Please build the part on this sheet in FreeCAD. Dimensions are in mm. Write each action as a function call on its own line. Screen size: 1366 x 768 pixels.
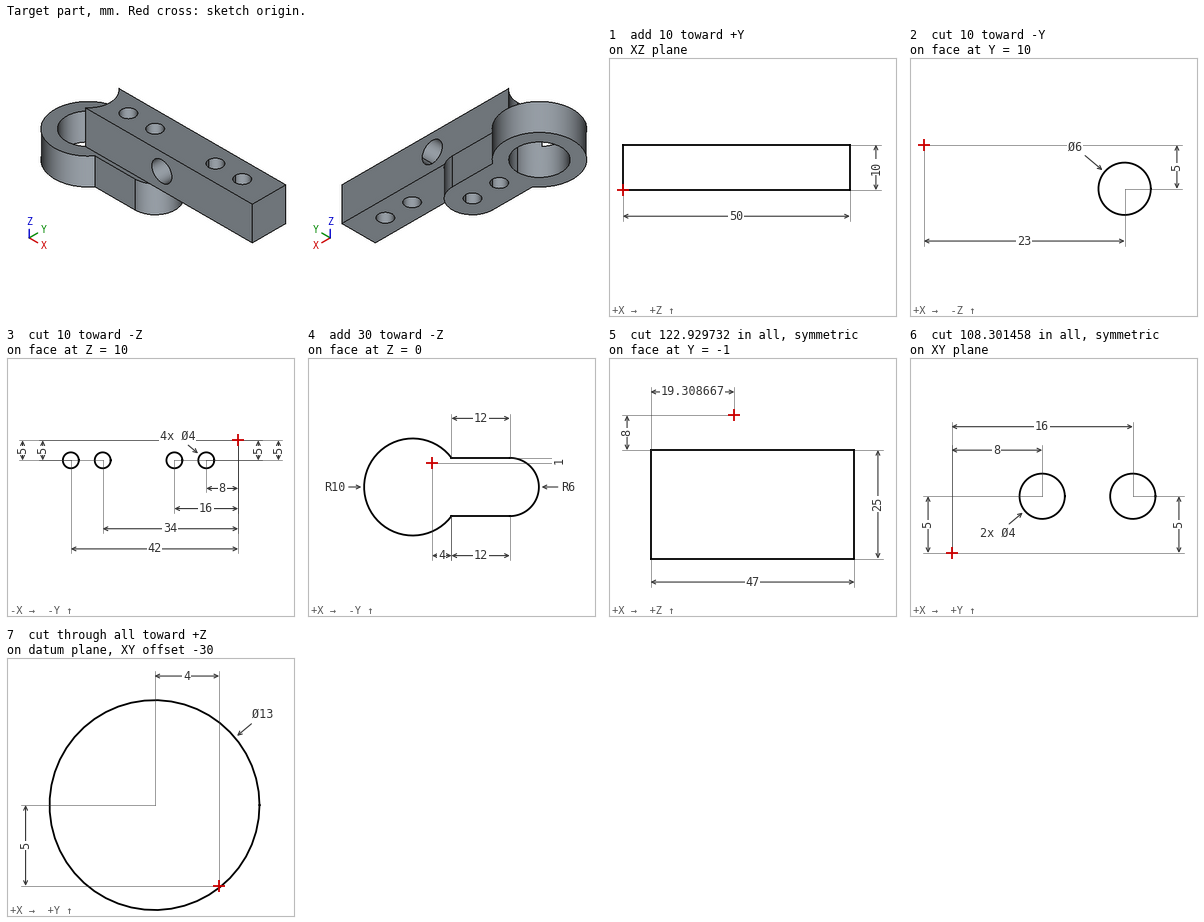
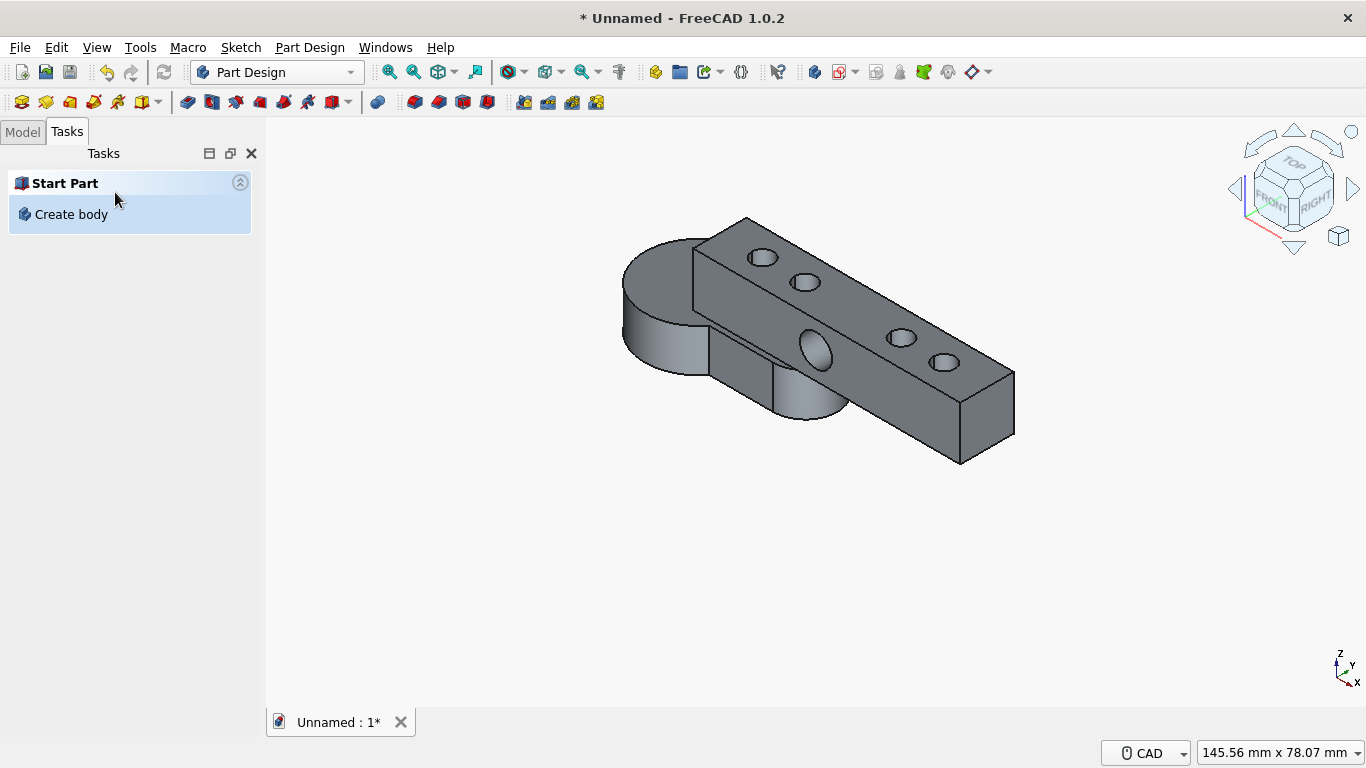
click(840, 72)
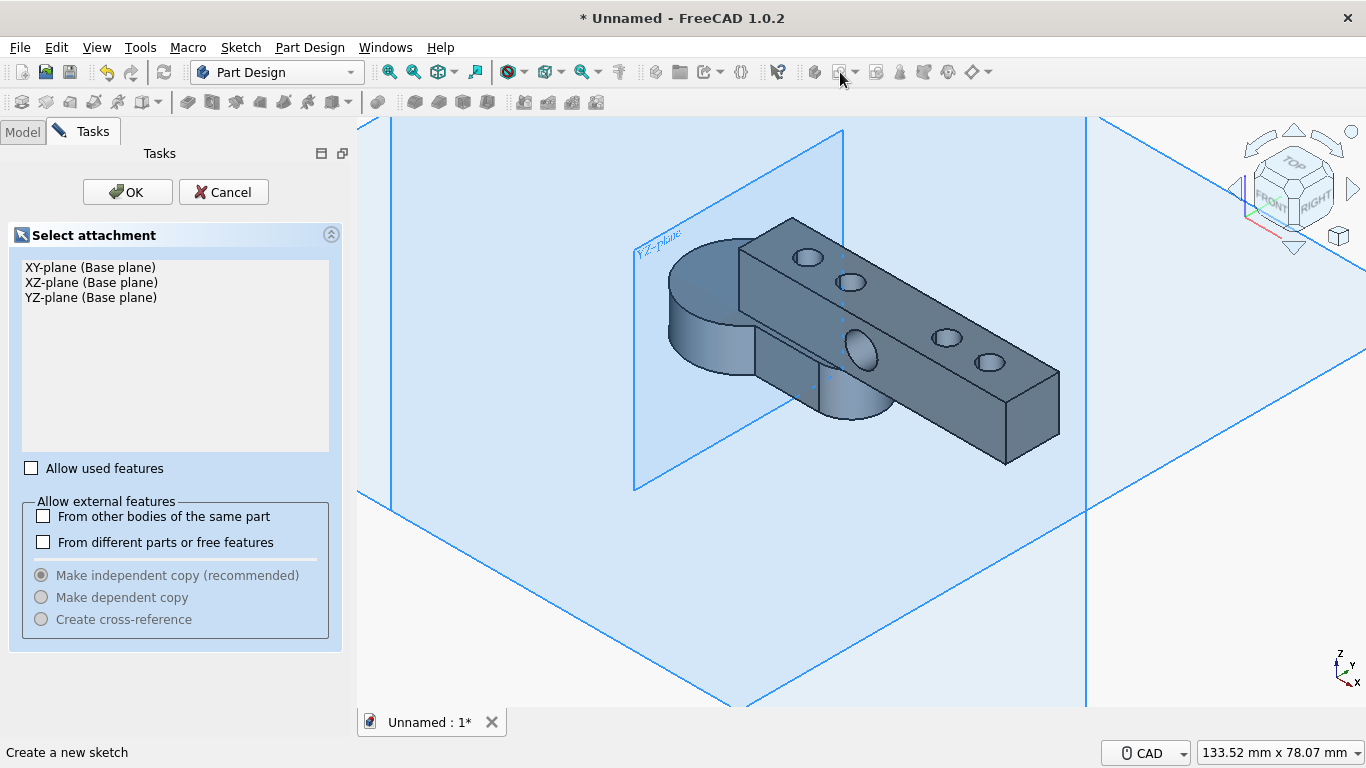
click(82, 268)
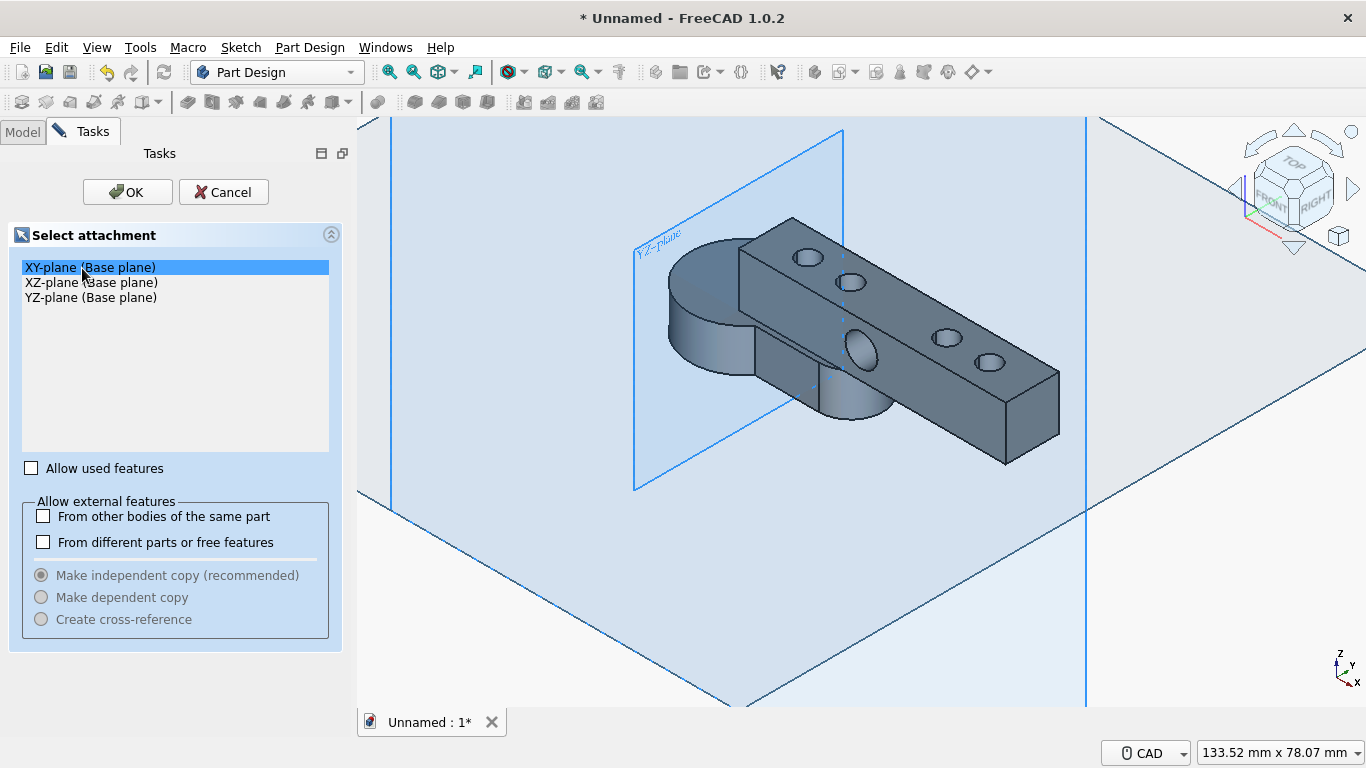
click(128, 192)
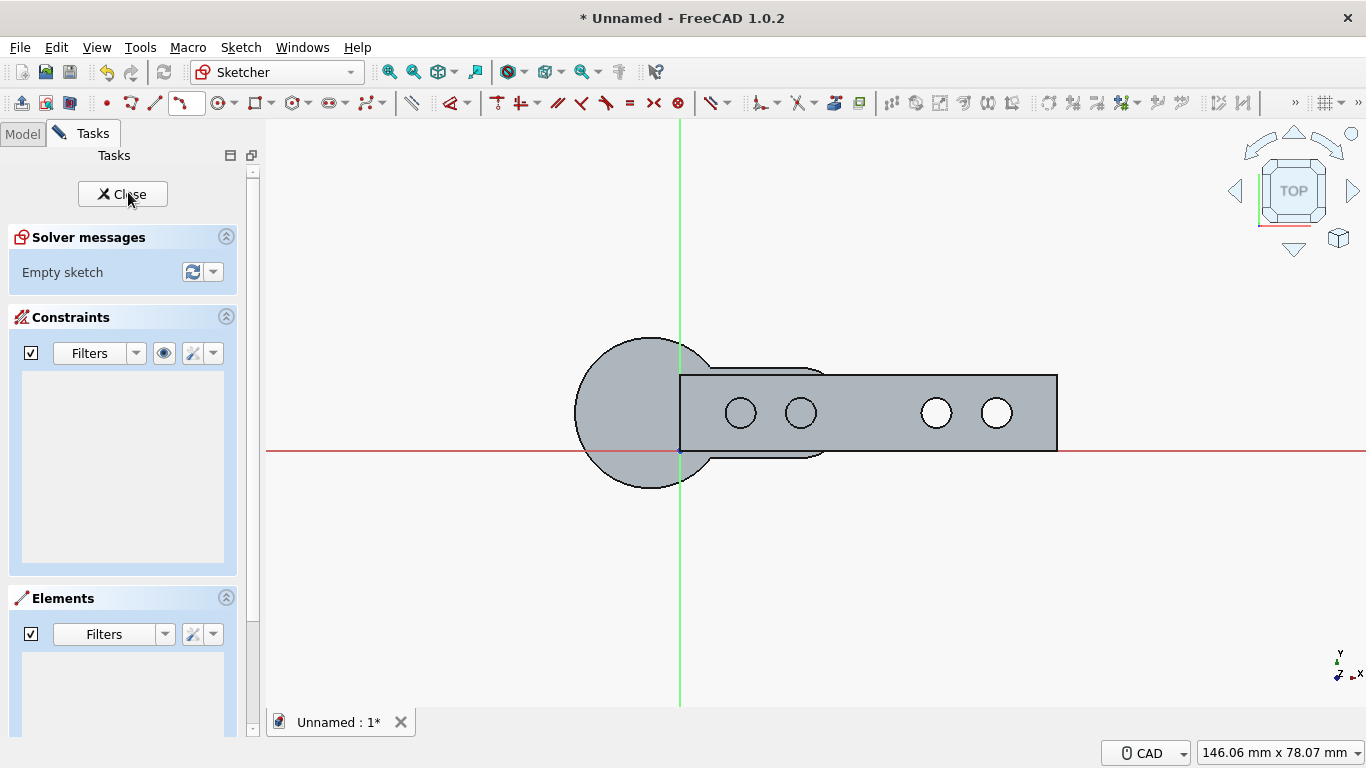
click(70, 104)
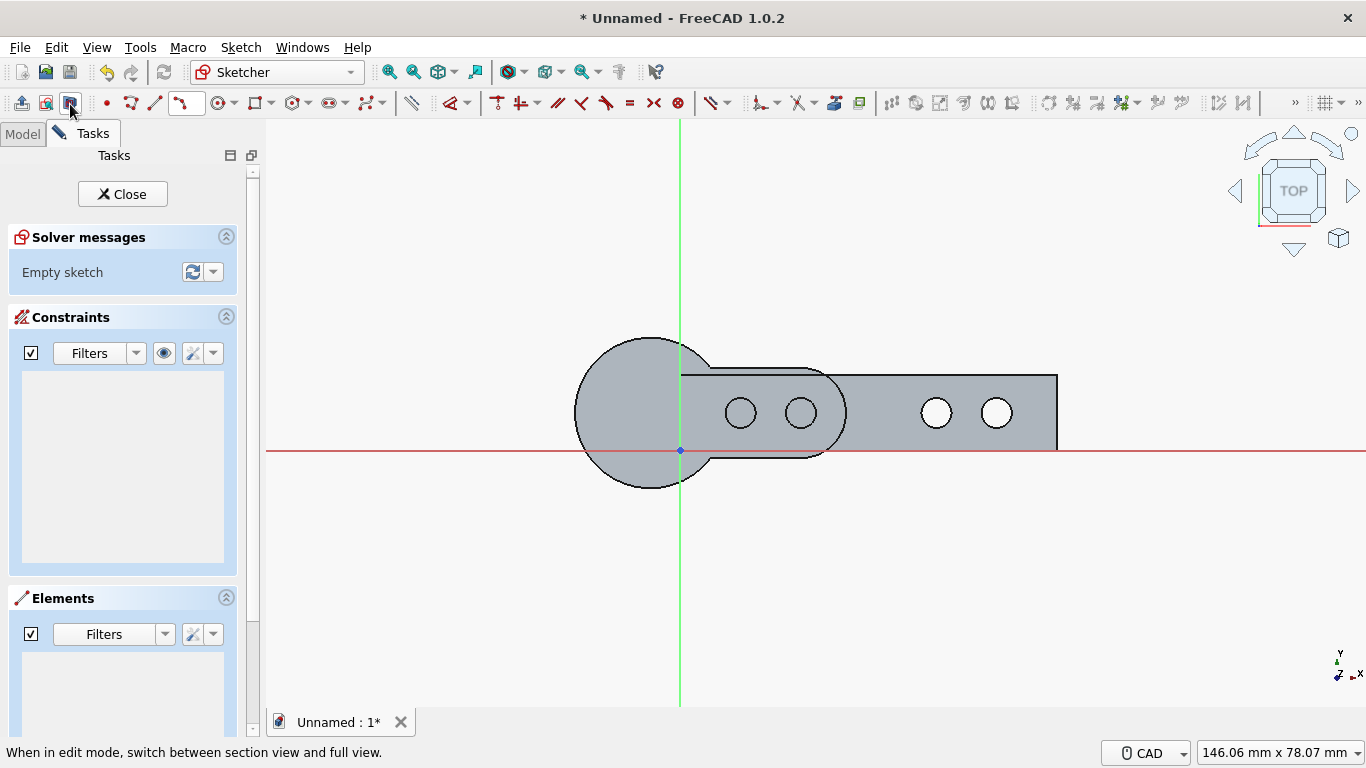
scroll(748, 427, up, 8)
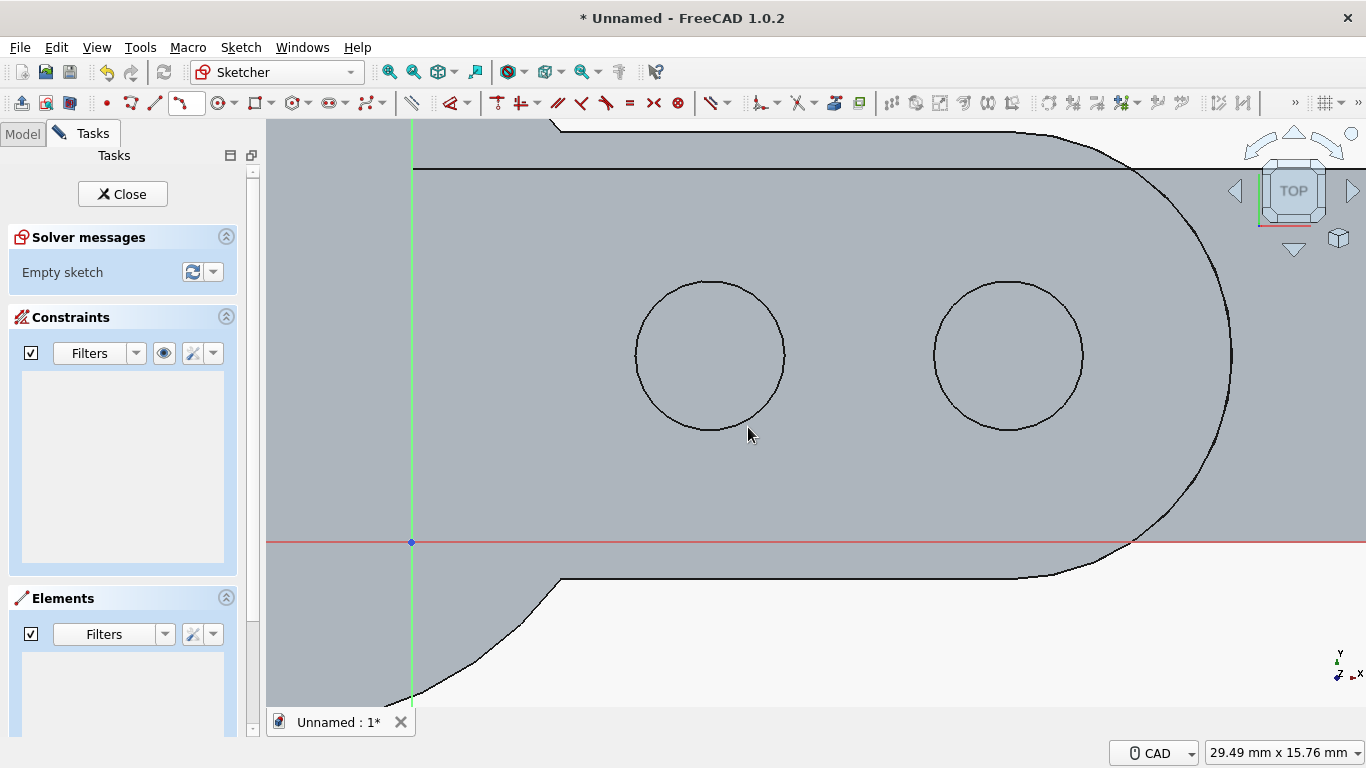
key(g)
key(c)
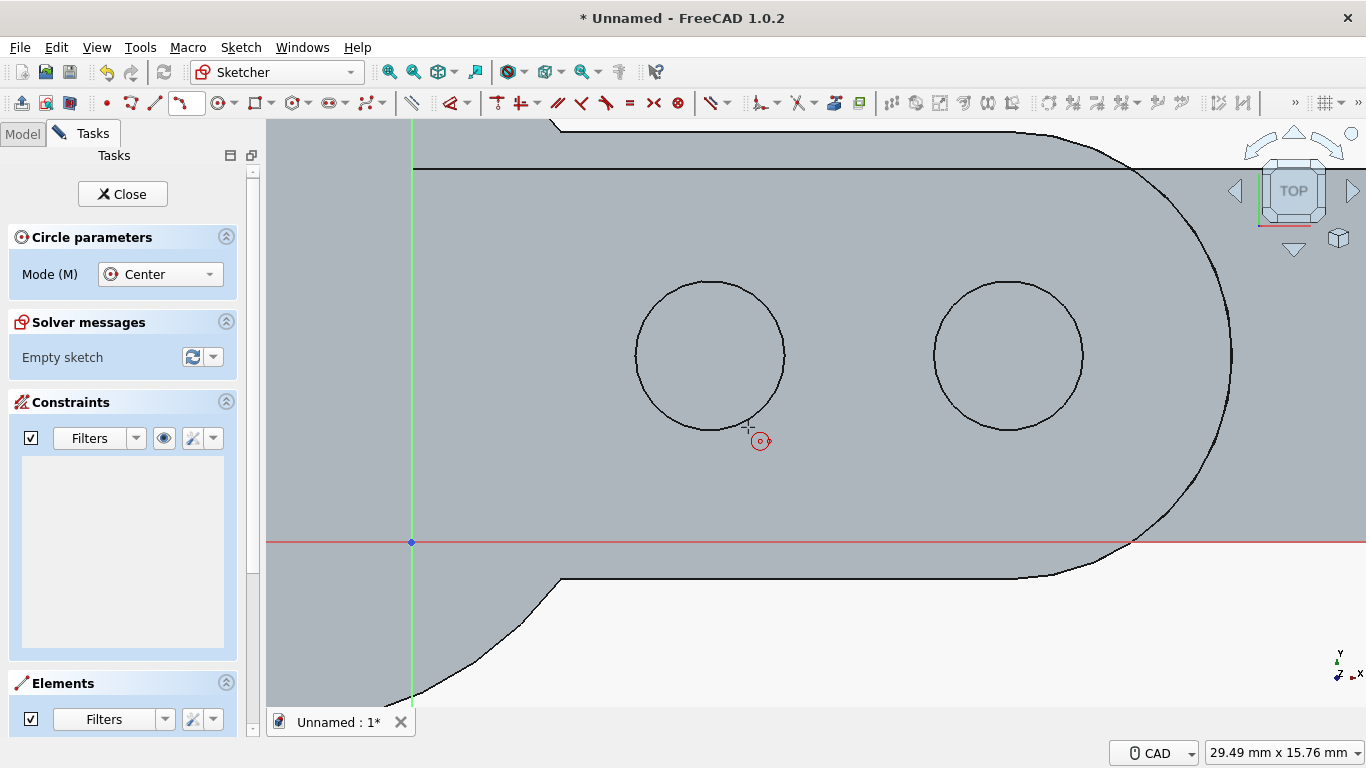
click(710, 356)
move(763, 303)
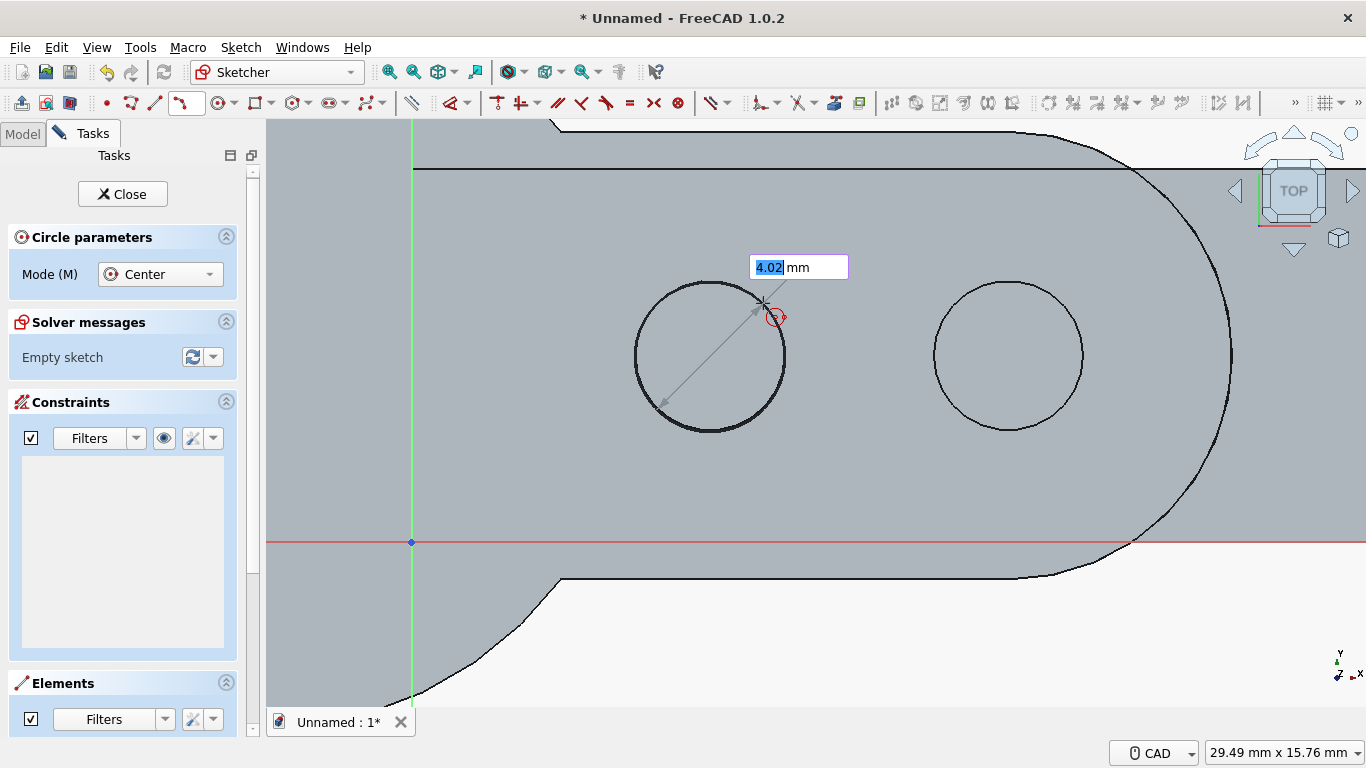
text(4)
key(Return)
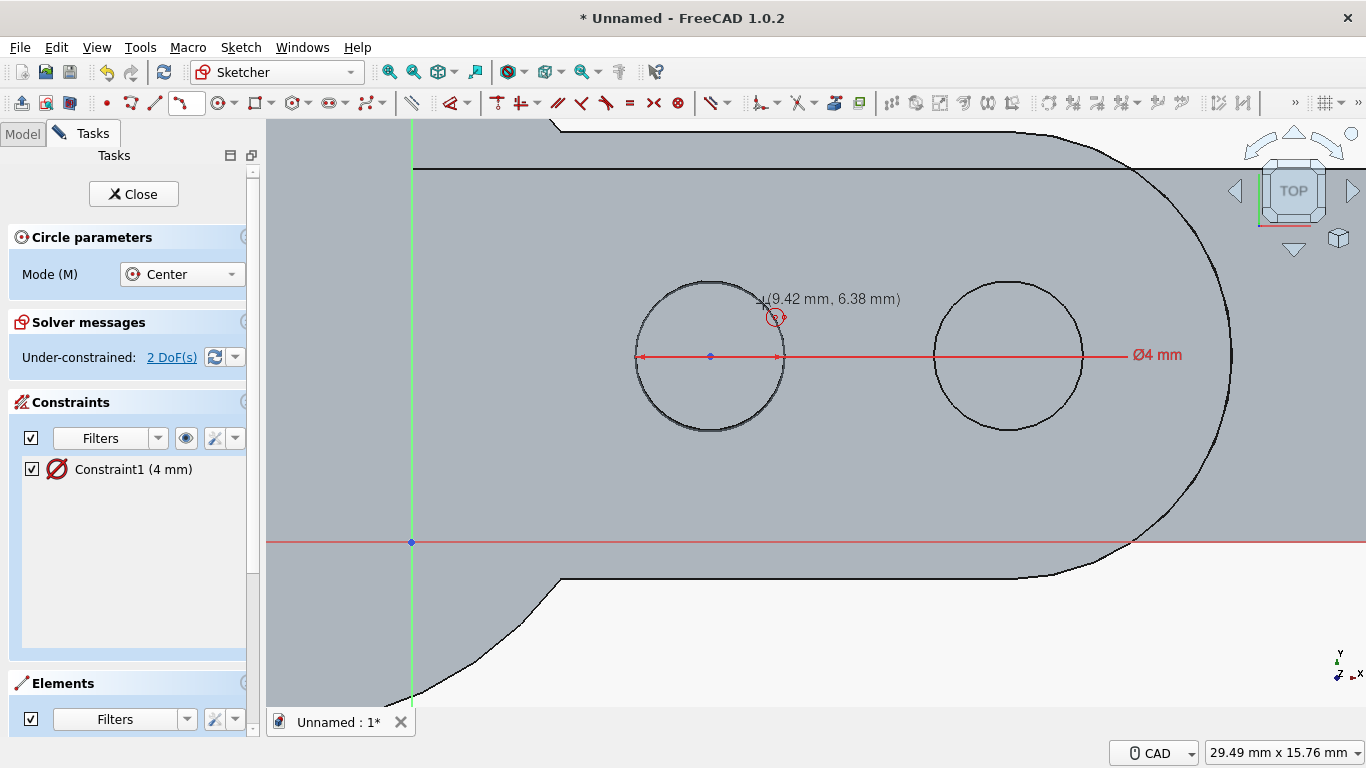
click(1008, 356)
move(1061, 303)